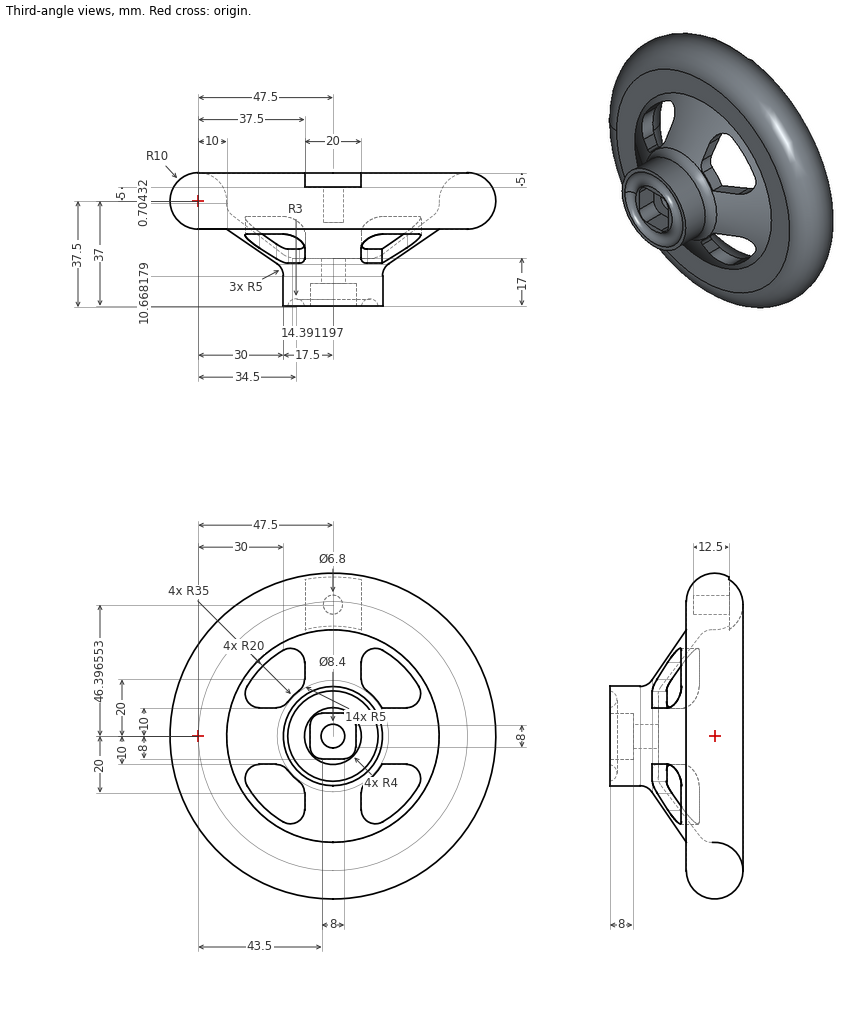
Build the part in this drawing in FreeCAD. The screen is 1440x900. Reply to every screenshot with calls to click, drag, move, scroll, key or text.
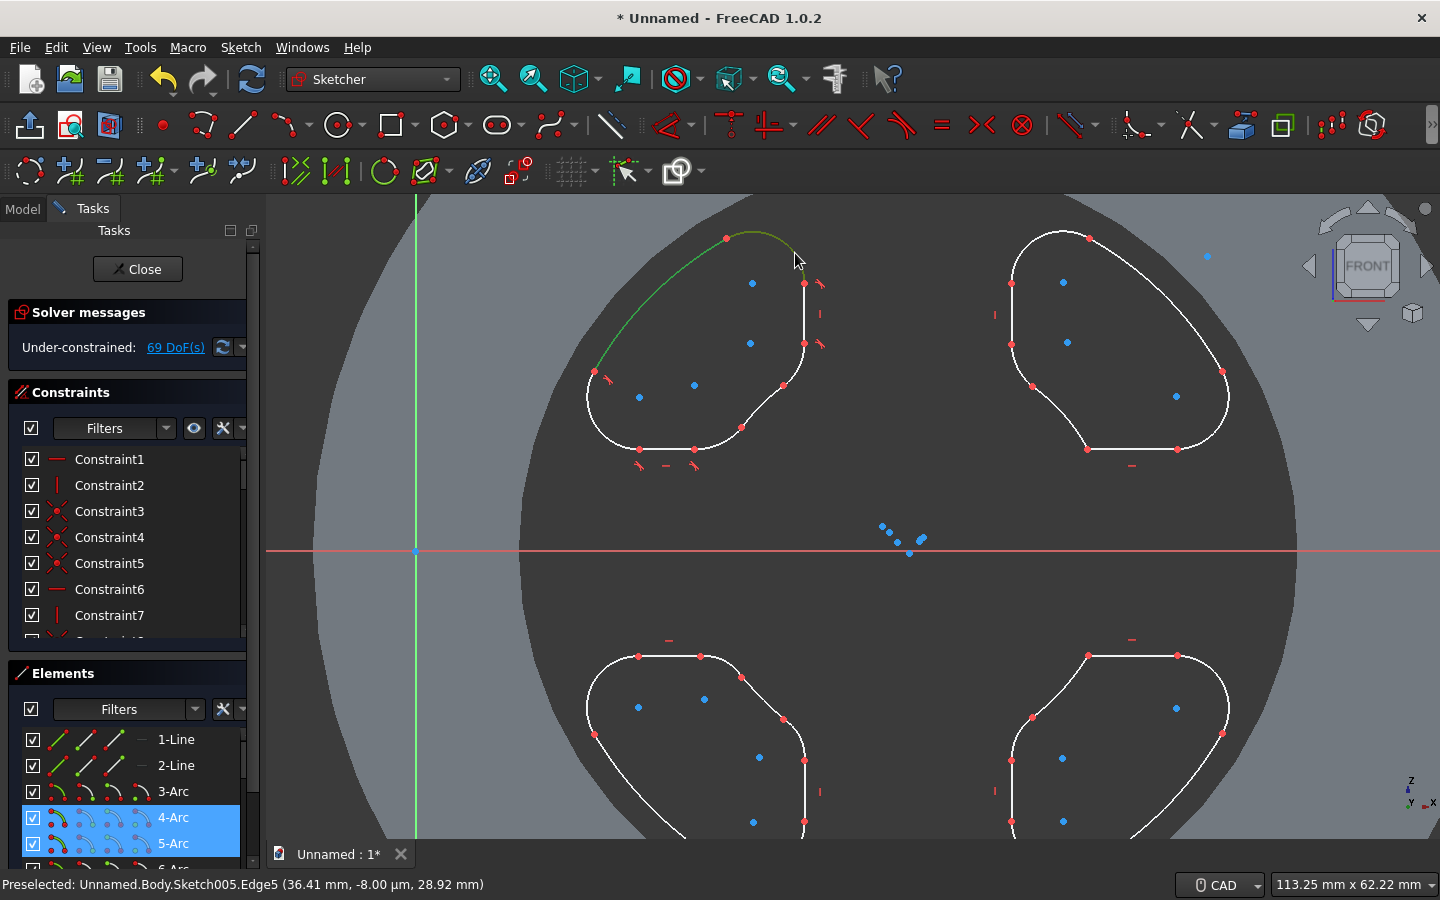
click(902, 126)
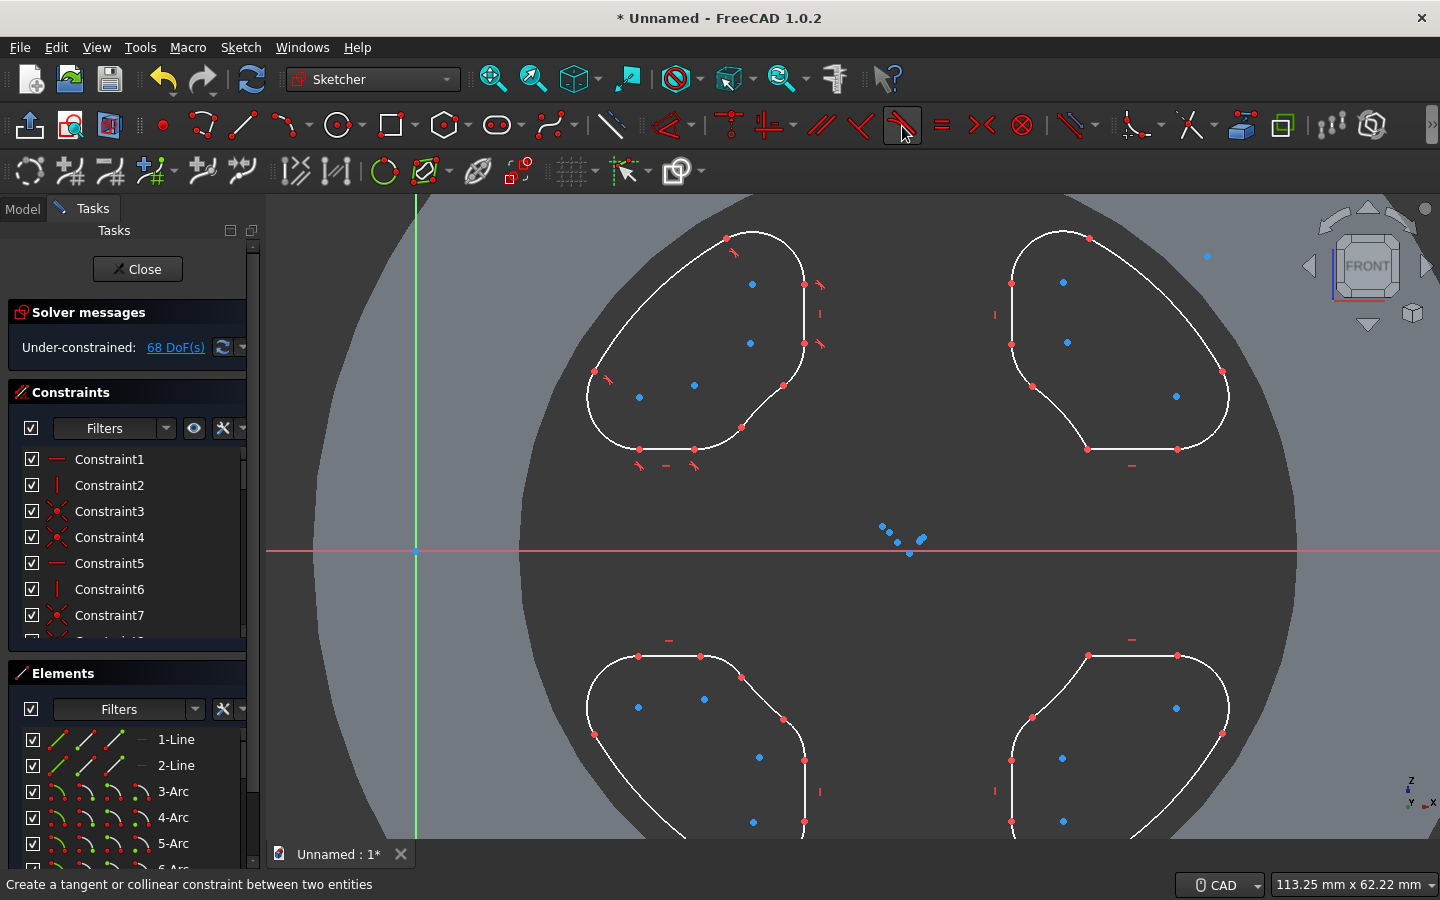
click(794, 375)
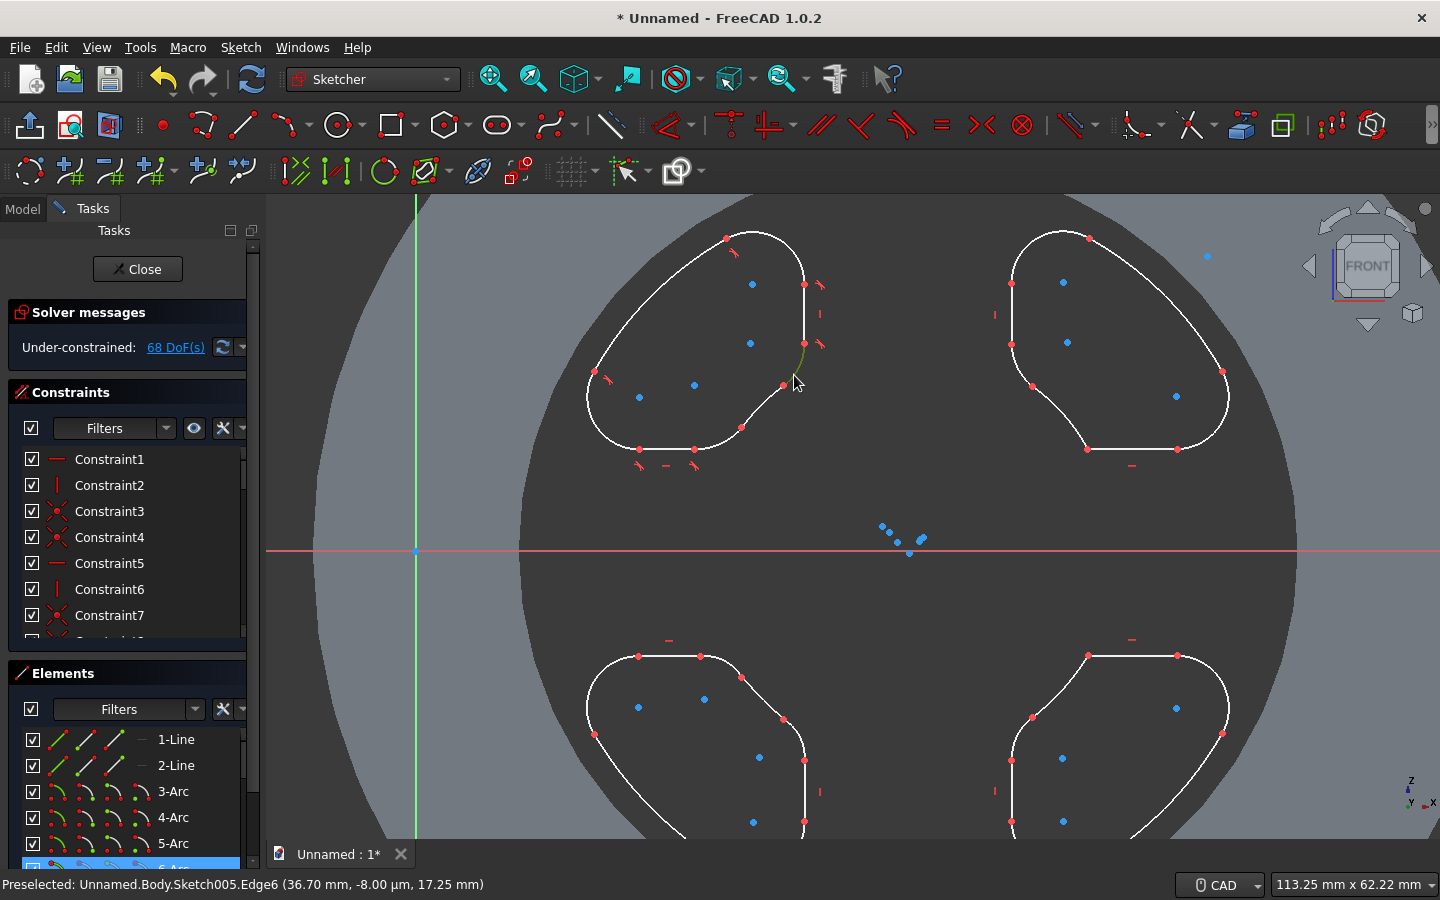
click(770, 397)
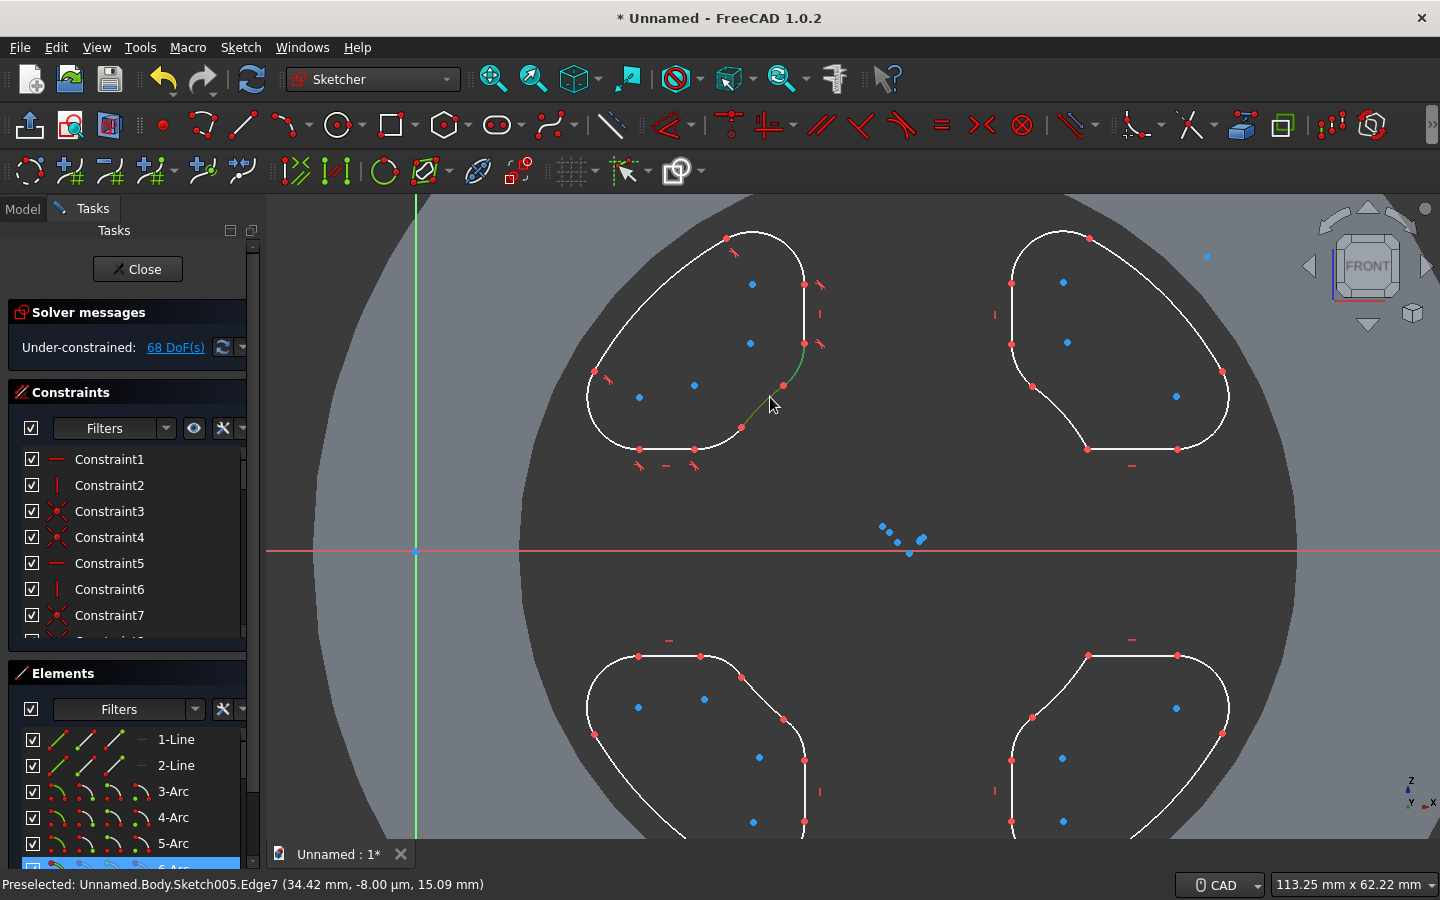
click(902, 126)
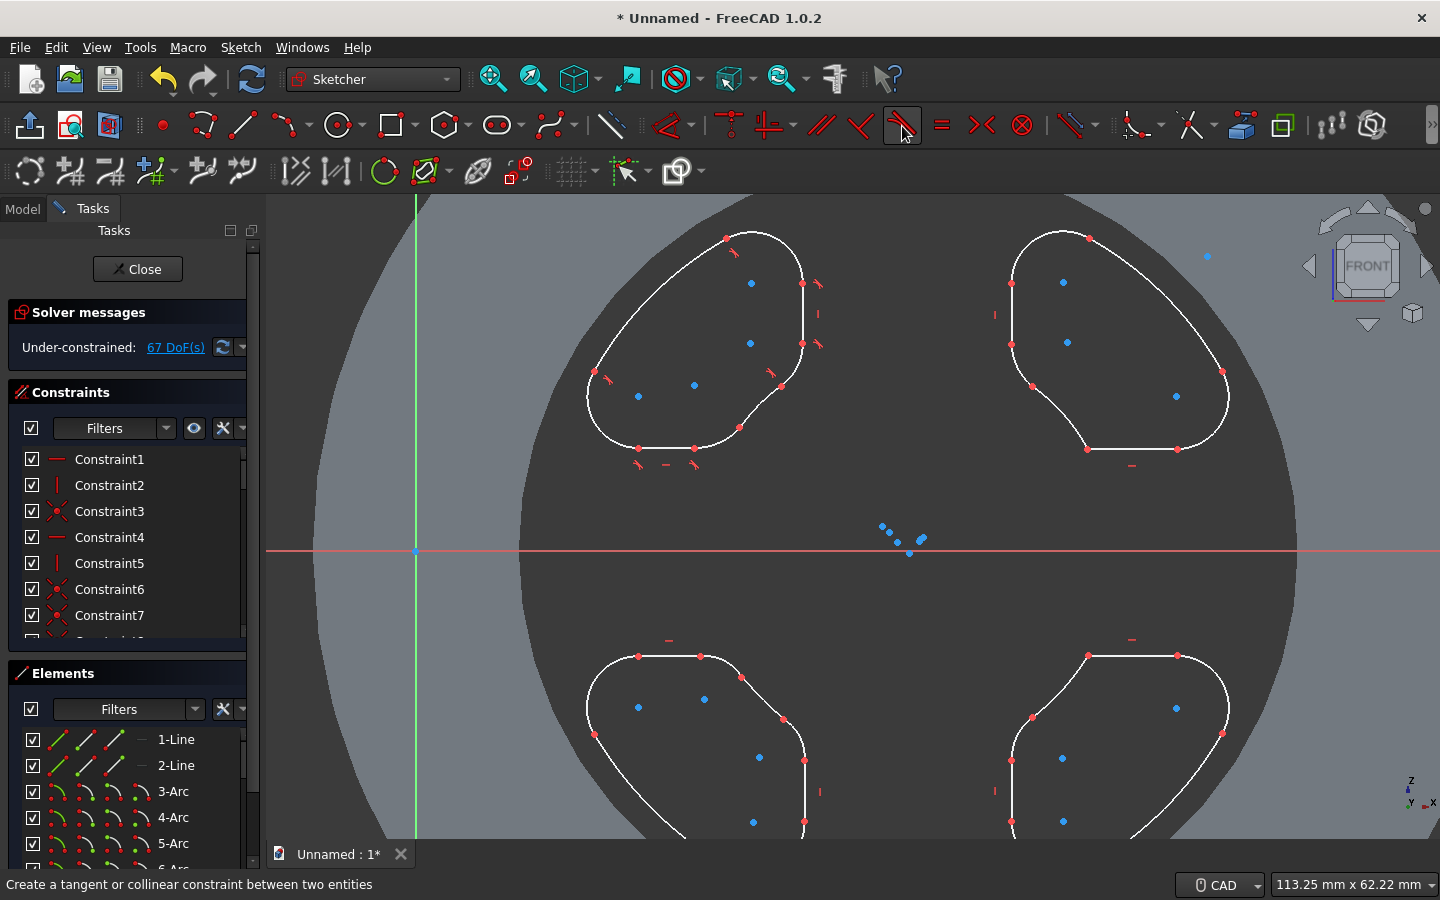
click(767, 397)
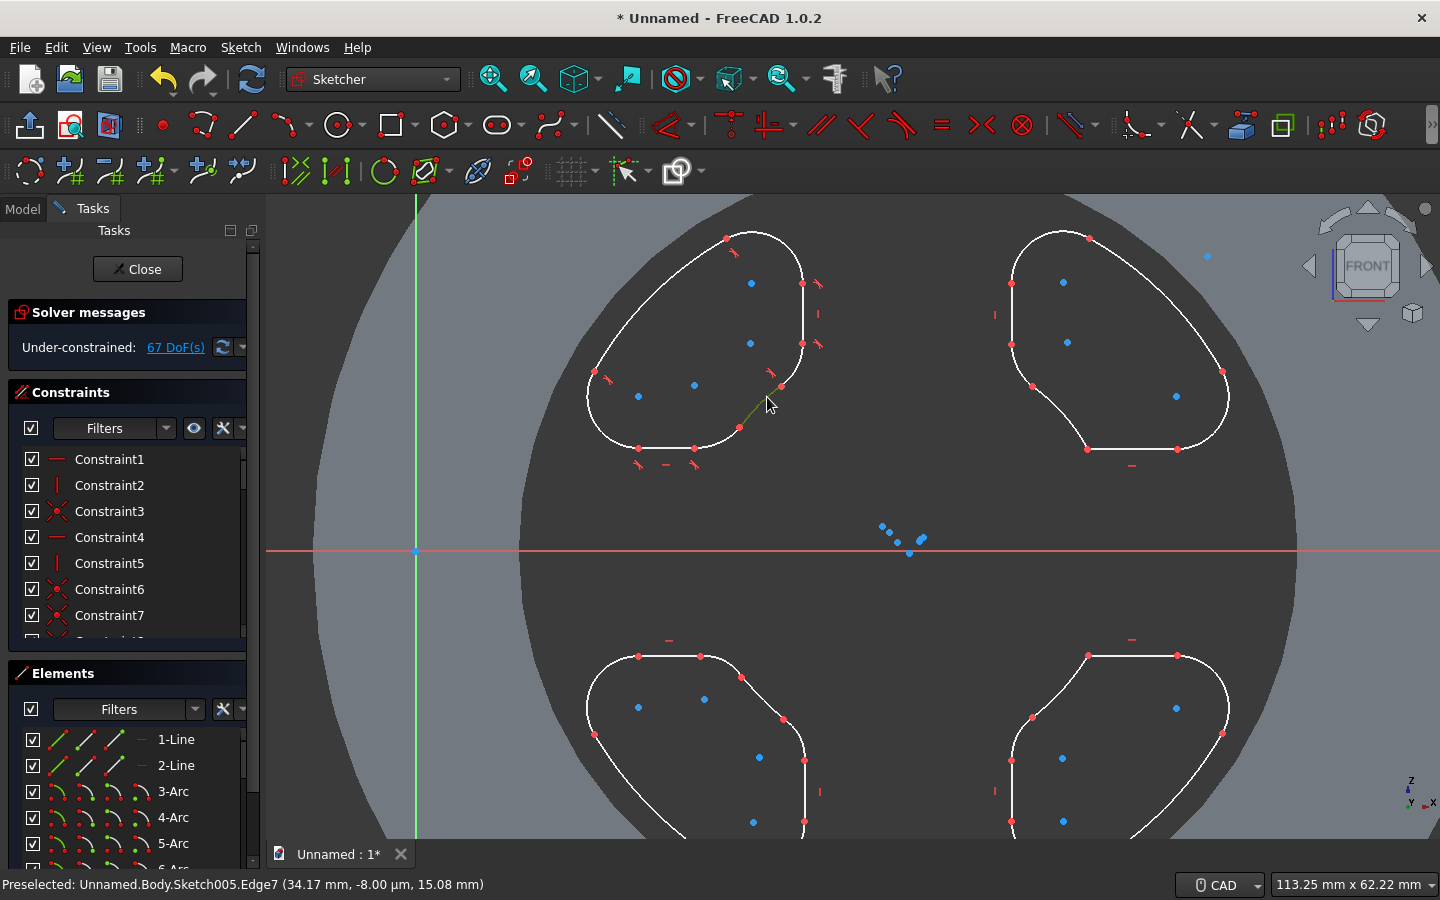
click(709, 446)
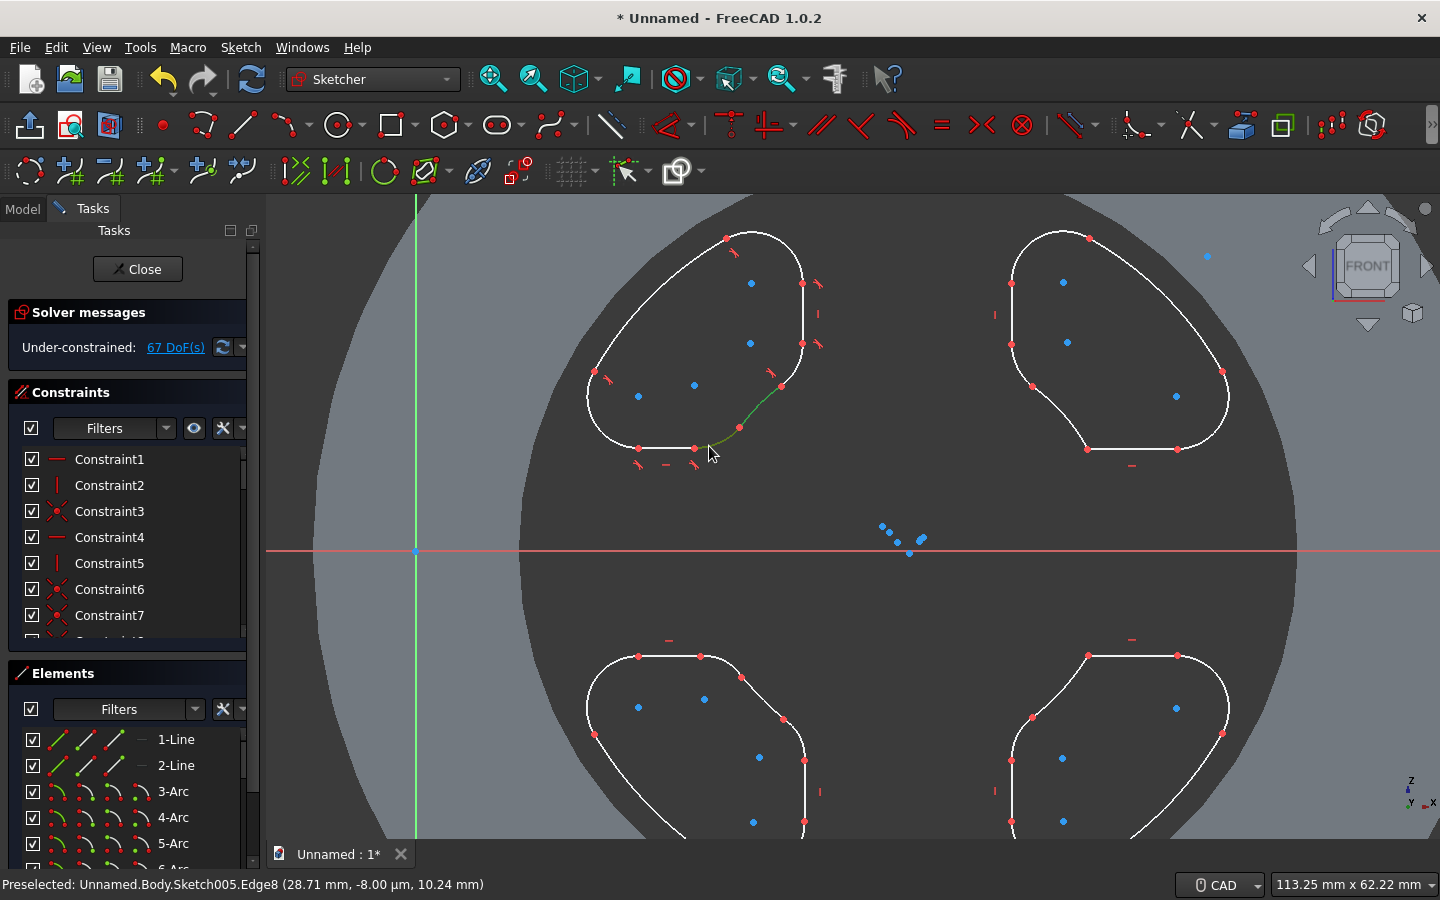
click(902, 126)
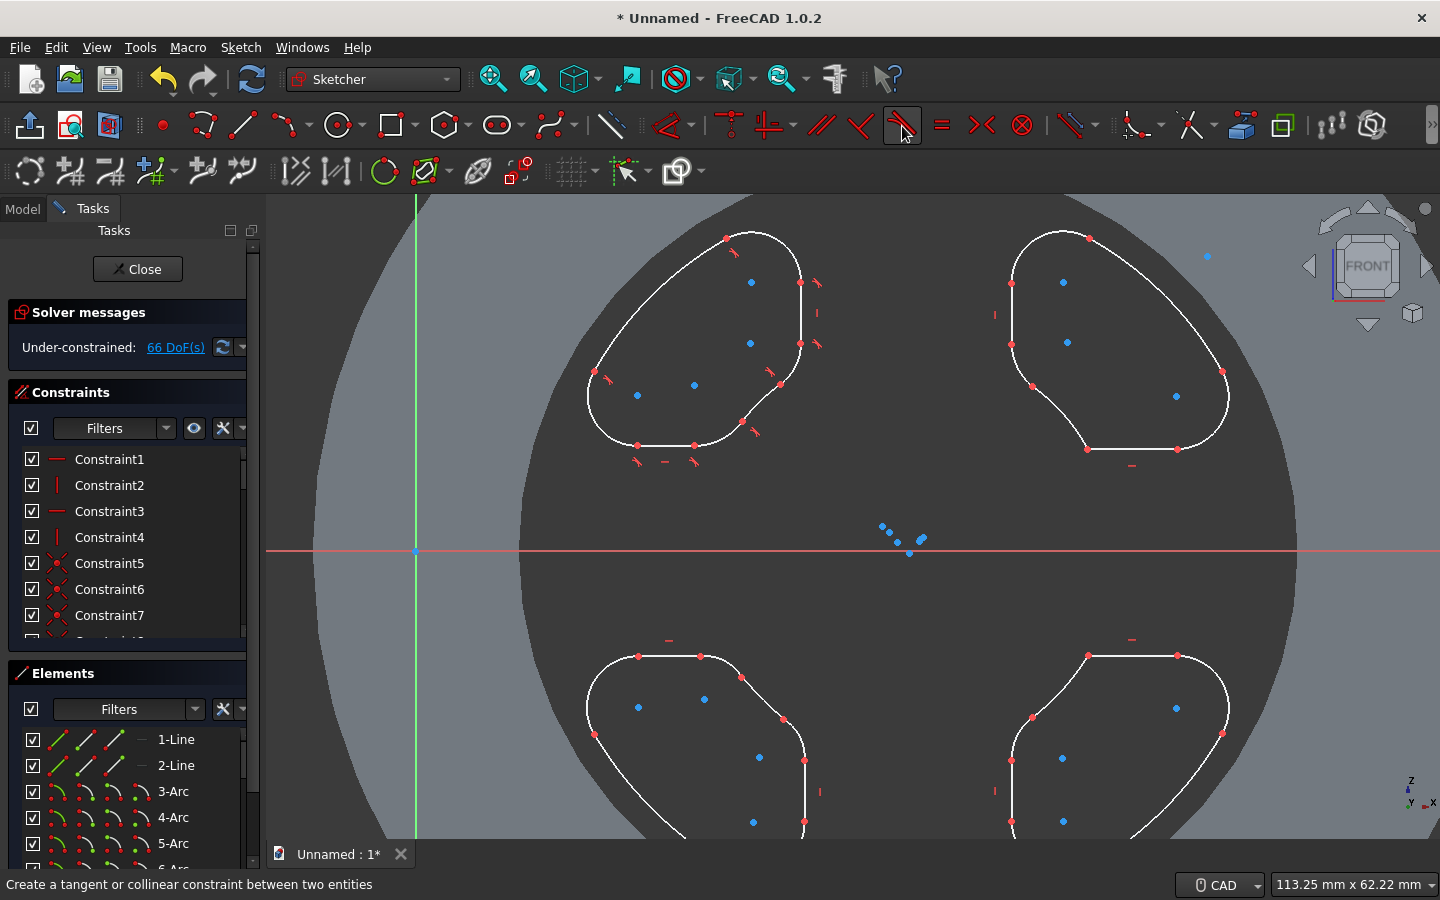
click(657, 656)